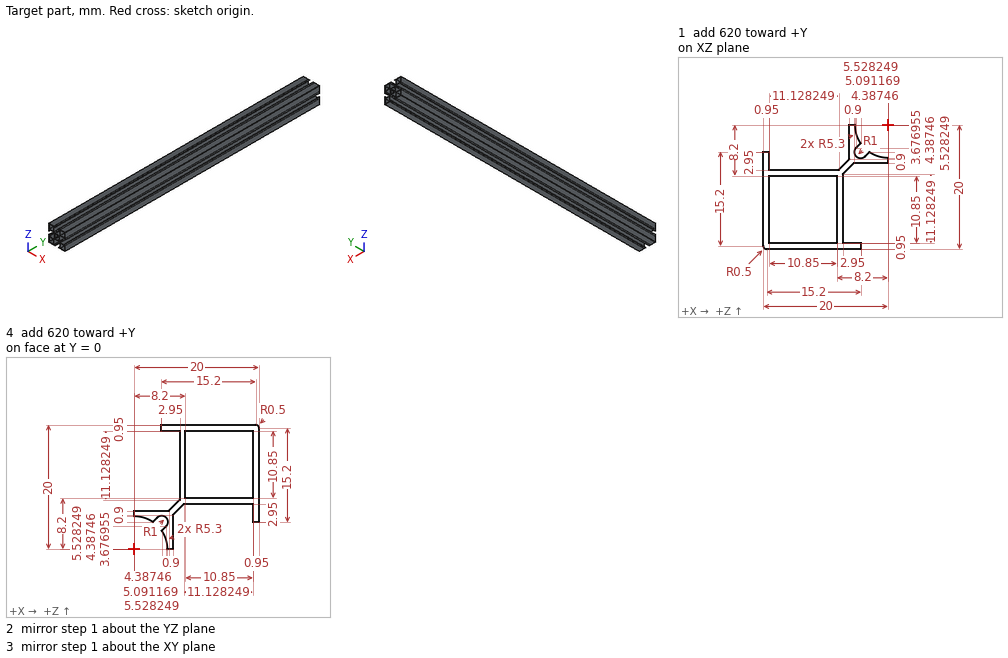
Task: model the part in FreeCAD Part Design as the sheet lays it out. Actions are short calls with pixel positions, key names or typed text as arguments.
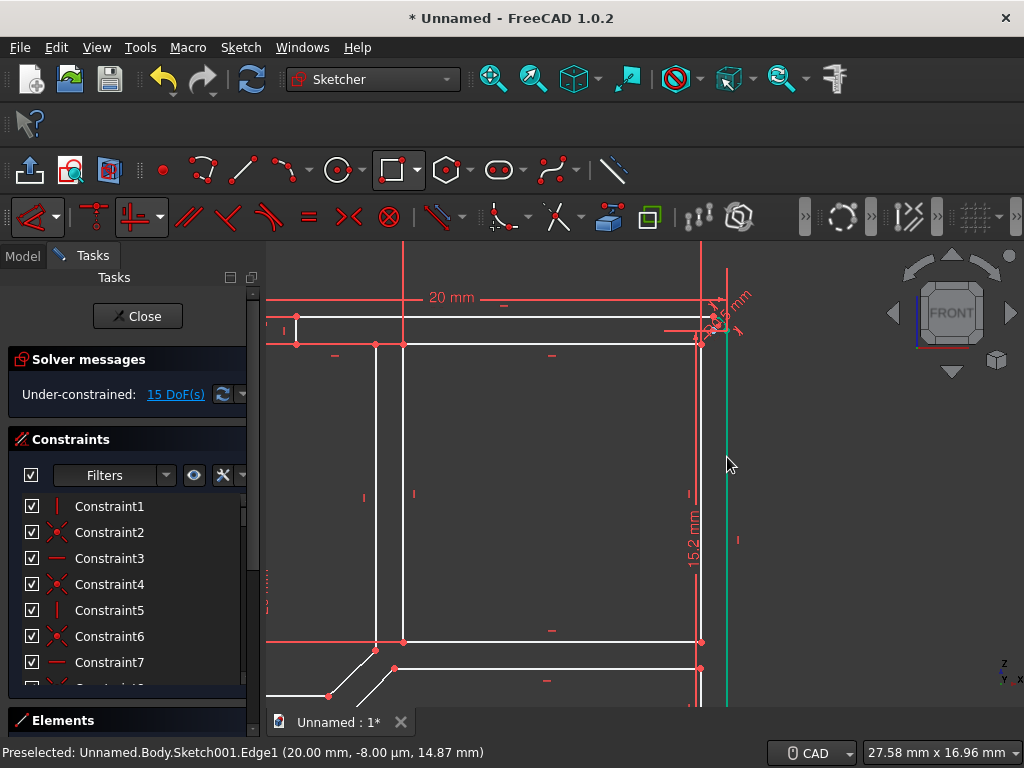
scroll(728, 331, down, 3)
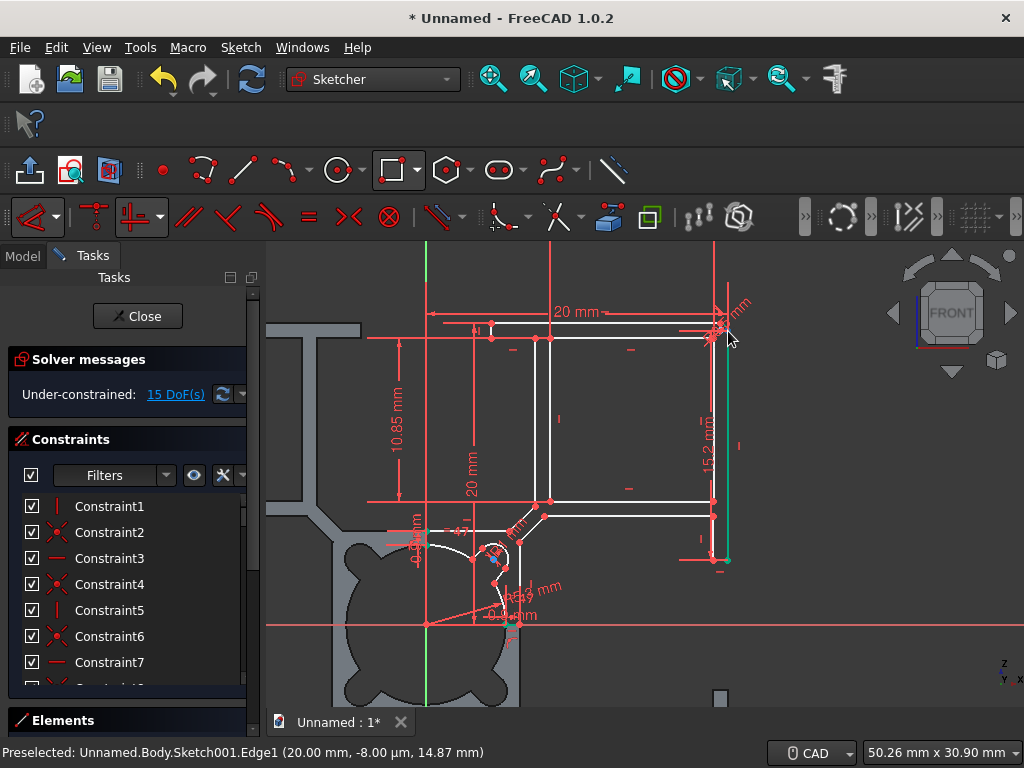
scroll(722, 560, up, 6)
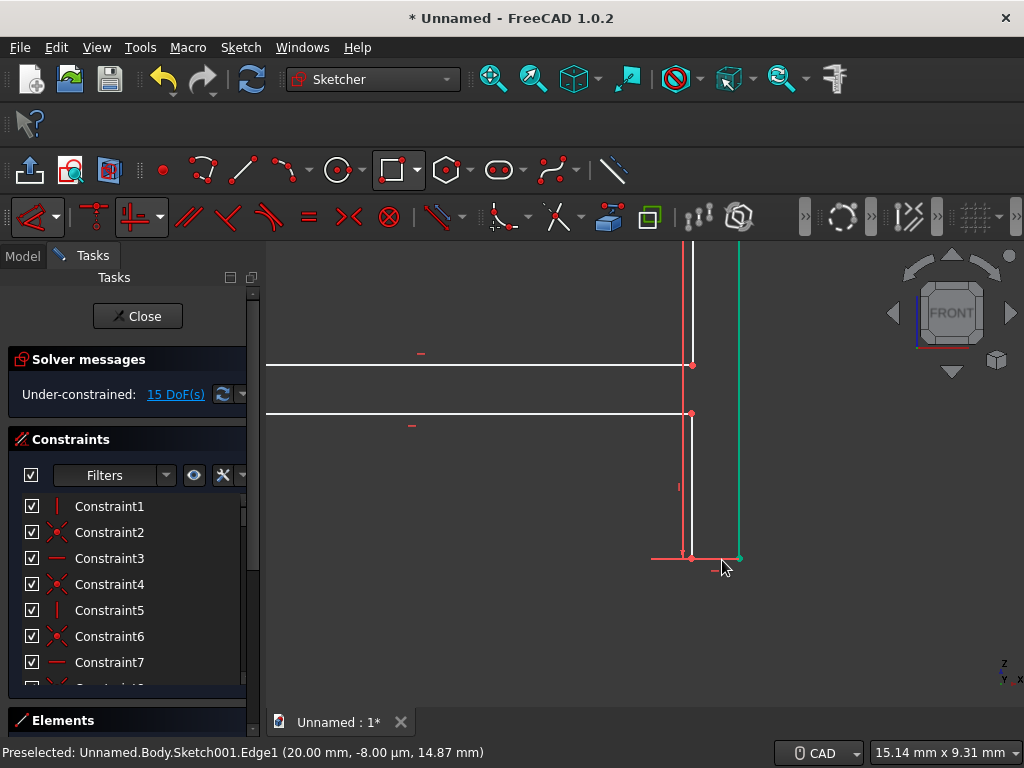
click(720, 559)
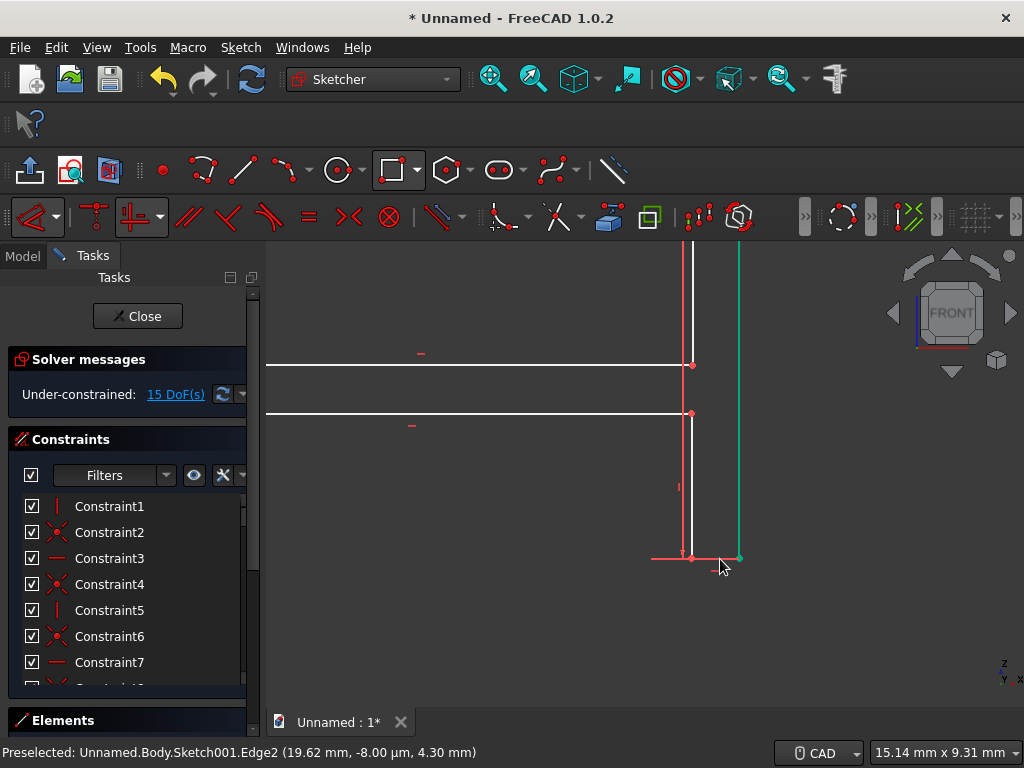
key(l)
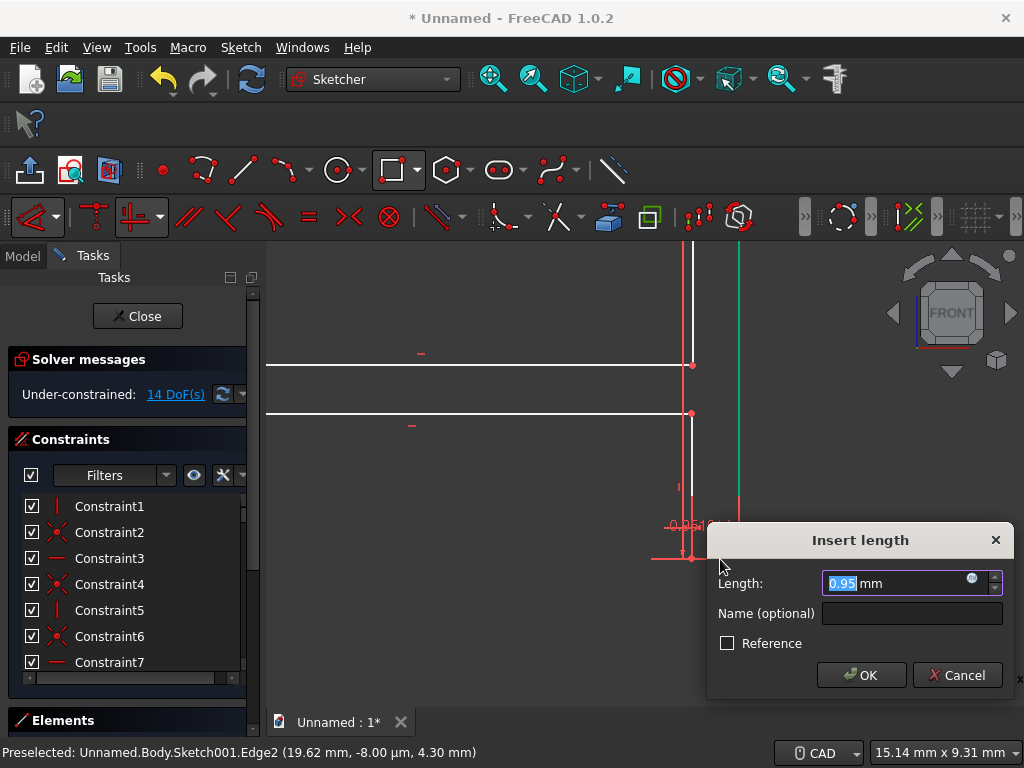
text(0.95)
key(Return)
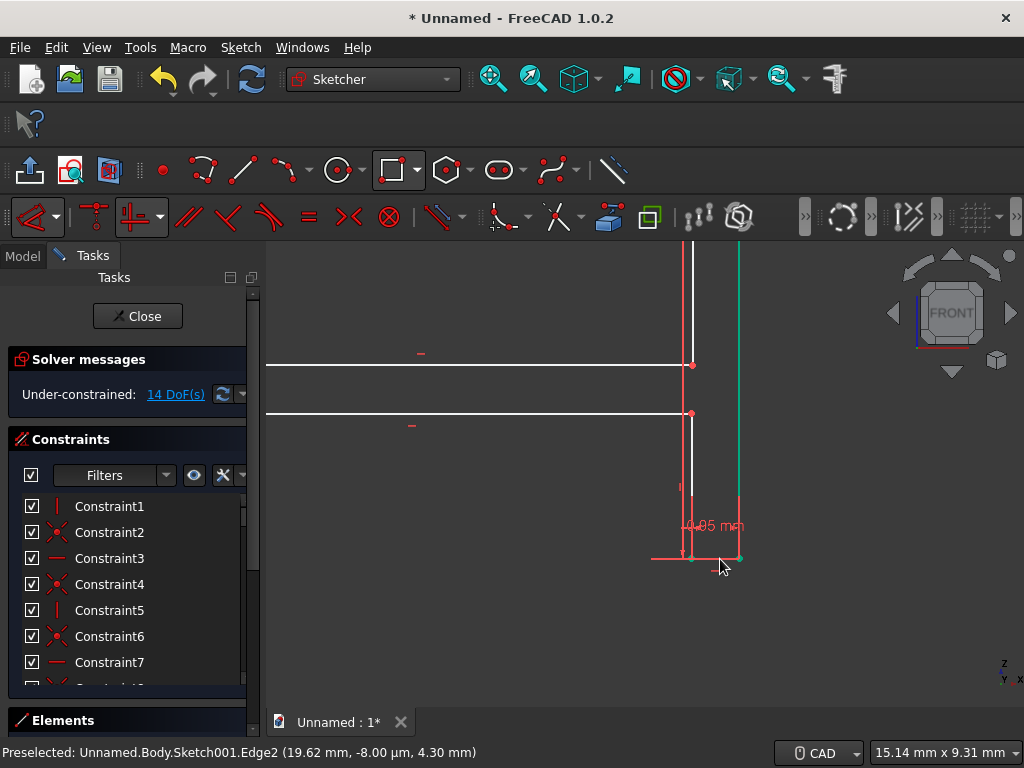
click(692, 515)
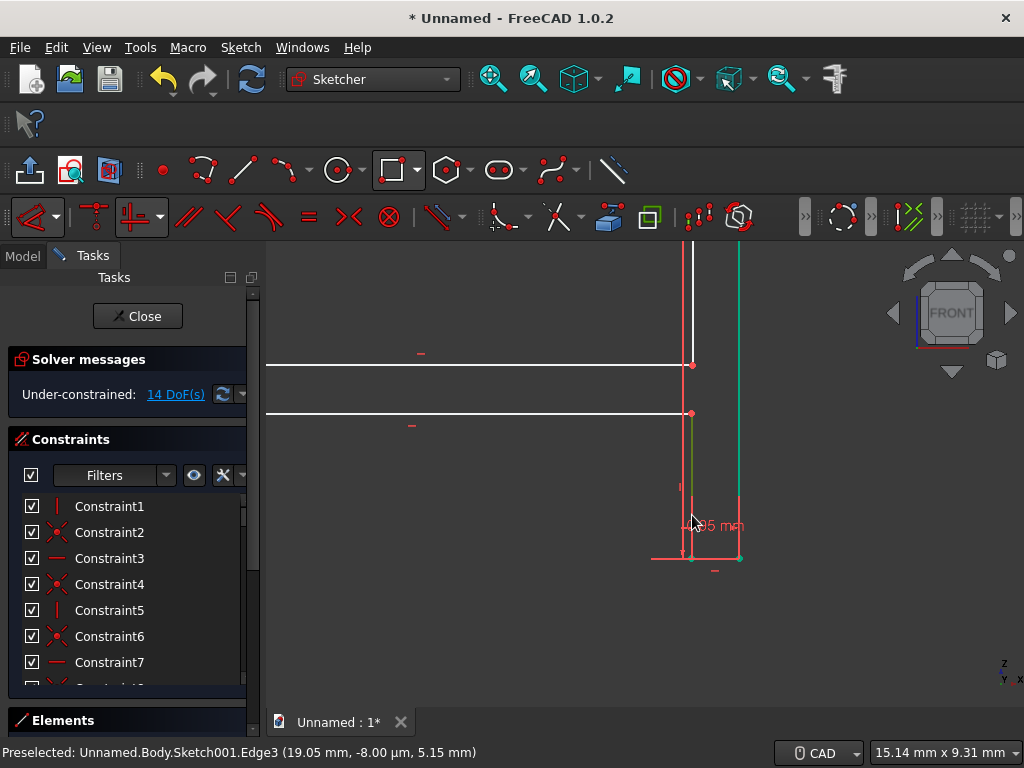
click(58, 218)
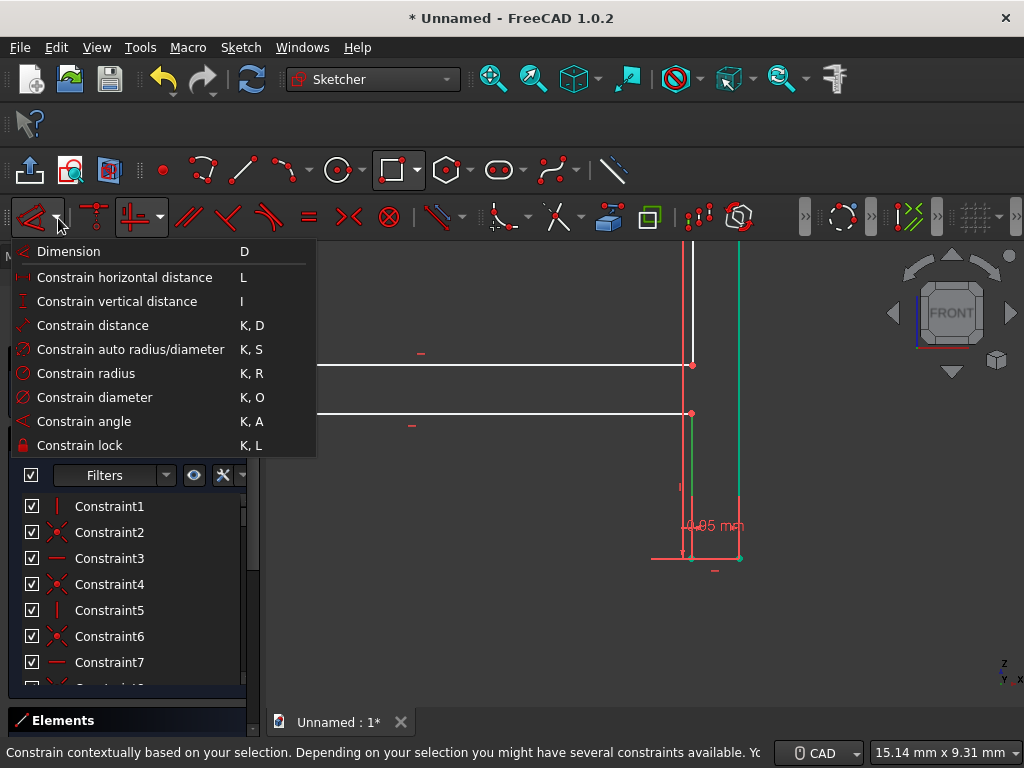
click(164, 301)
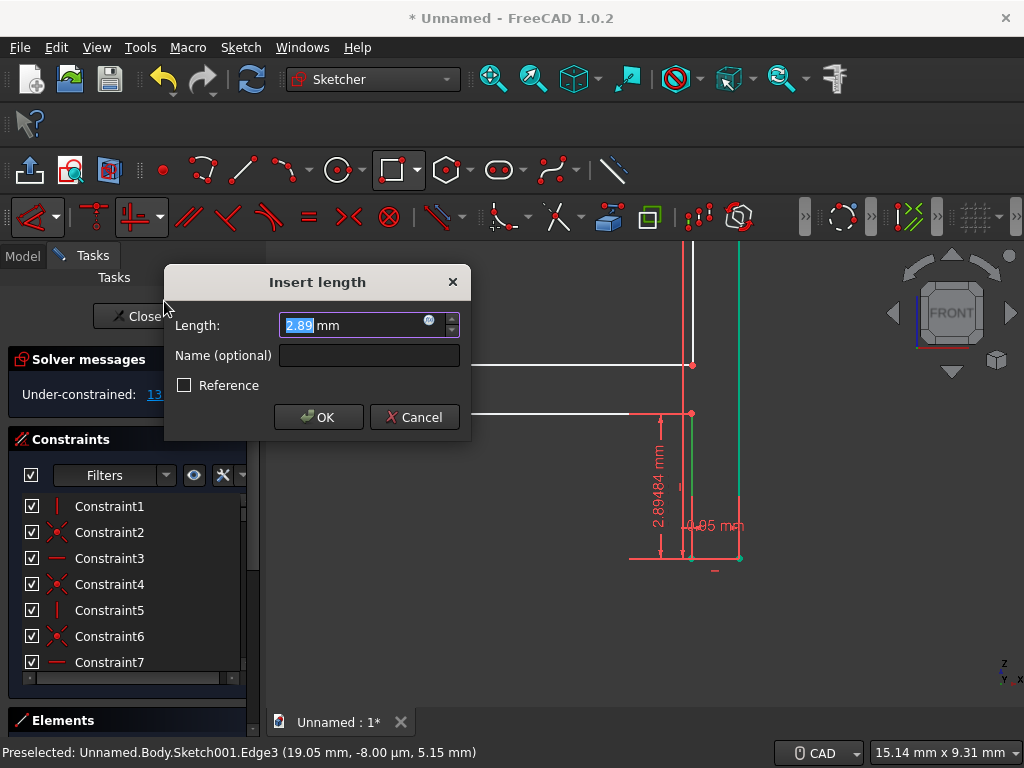
text(2.95)
key(Return)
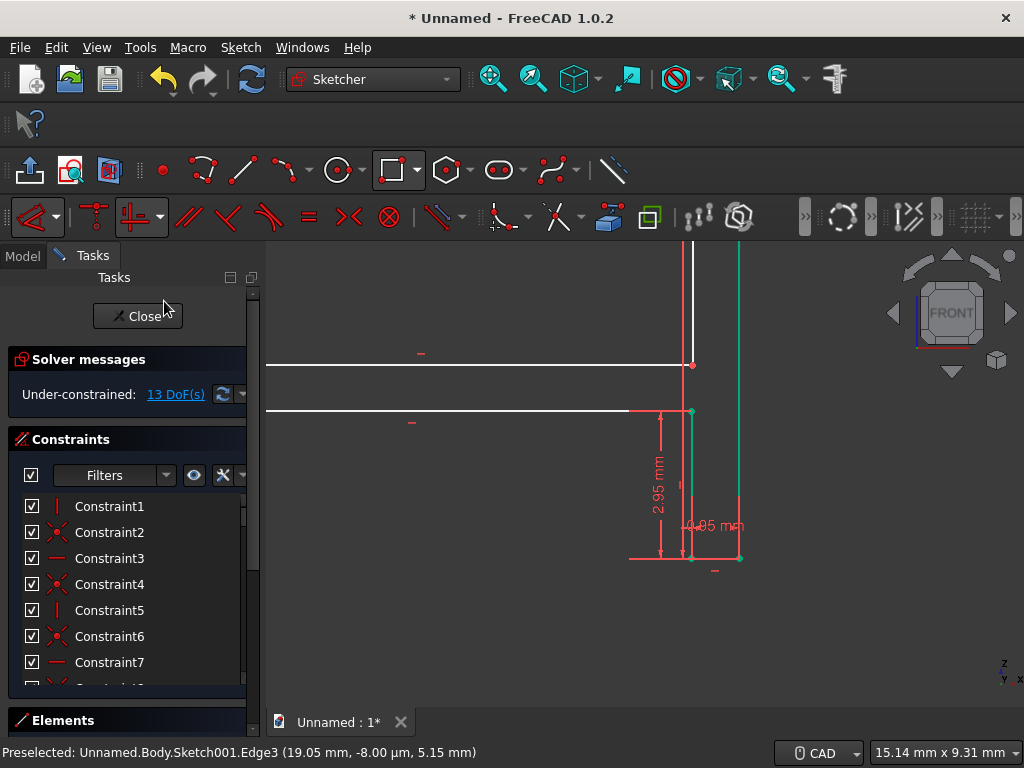
scroll(722, 560, down, 6)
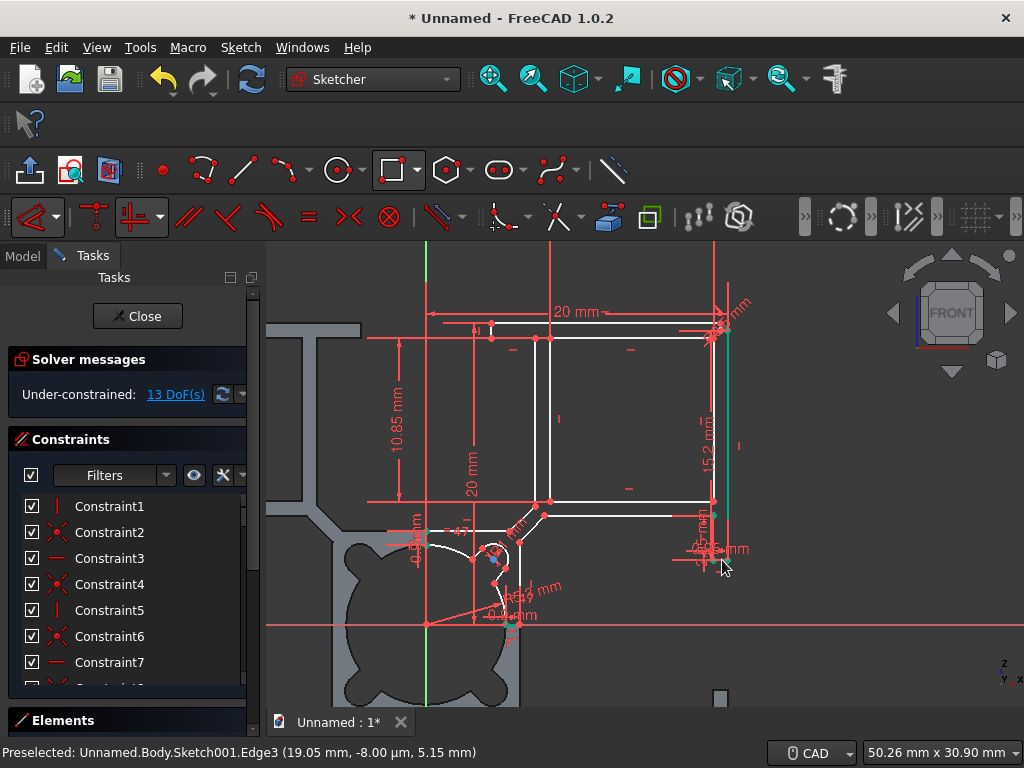
click(522, 338)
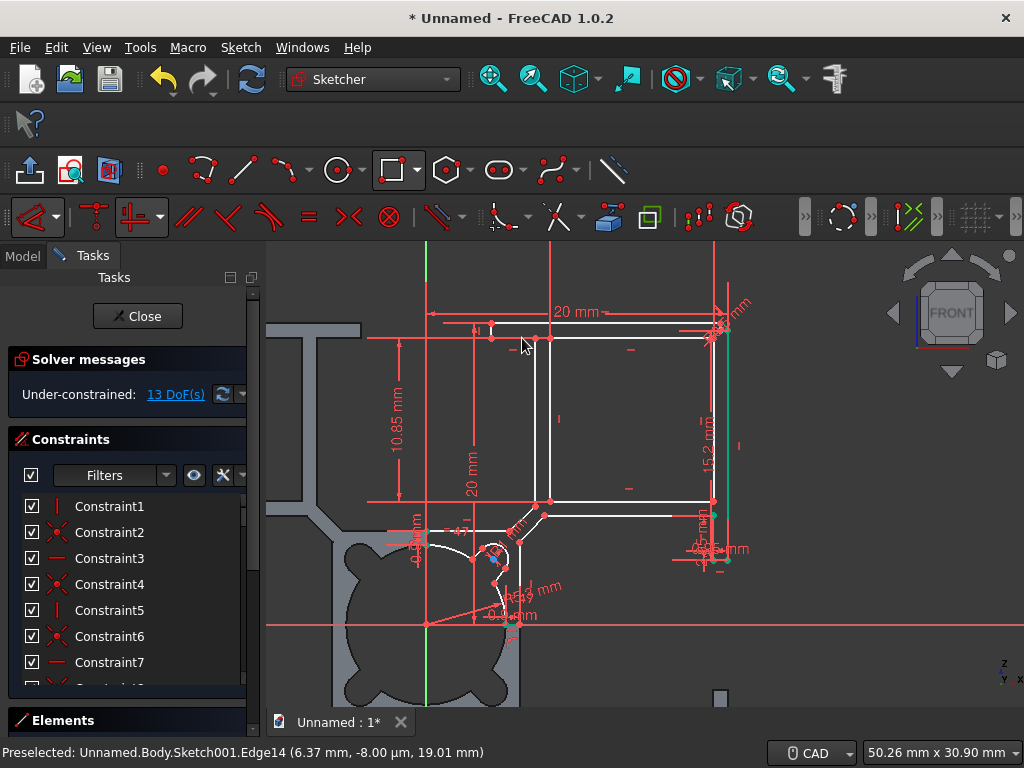
key(l)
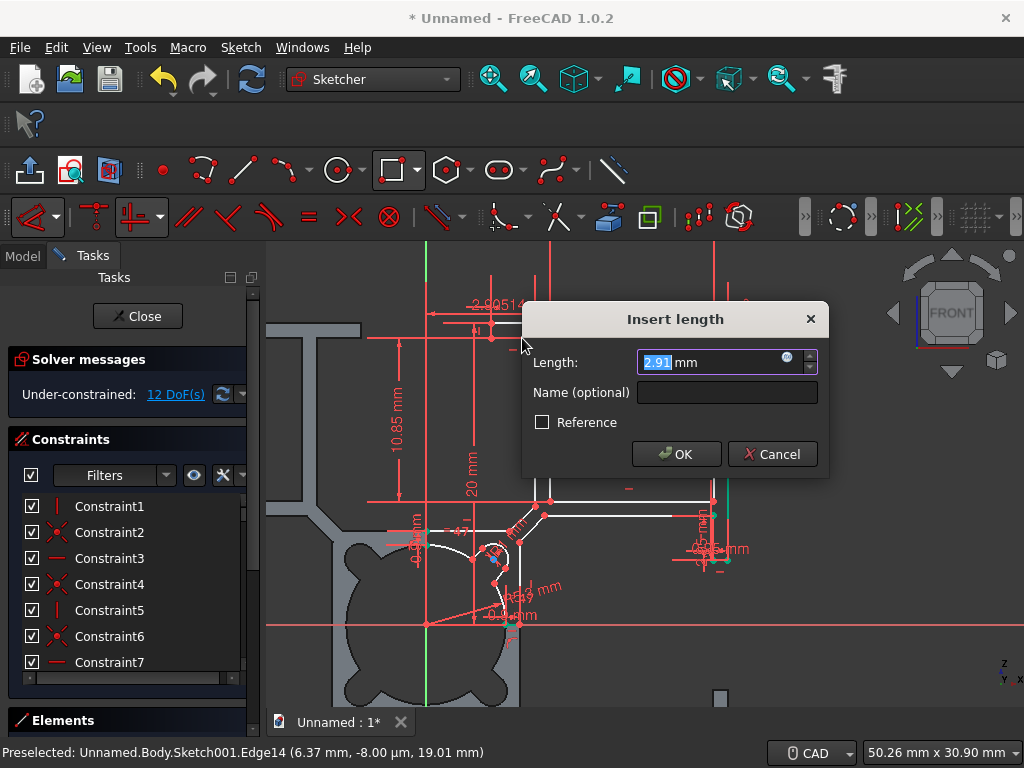
text(2.95)
key(Return)